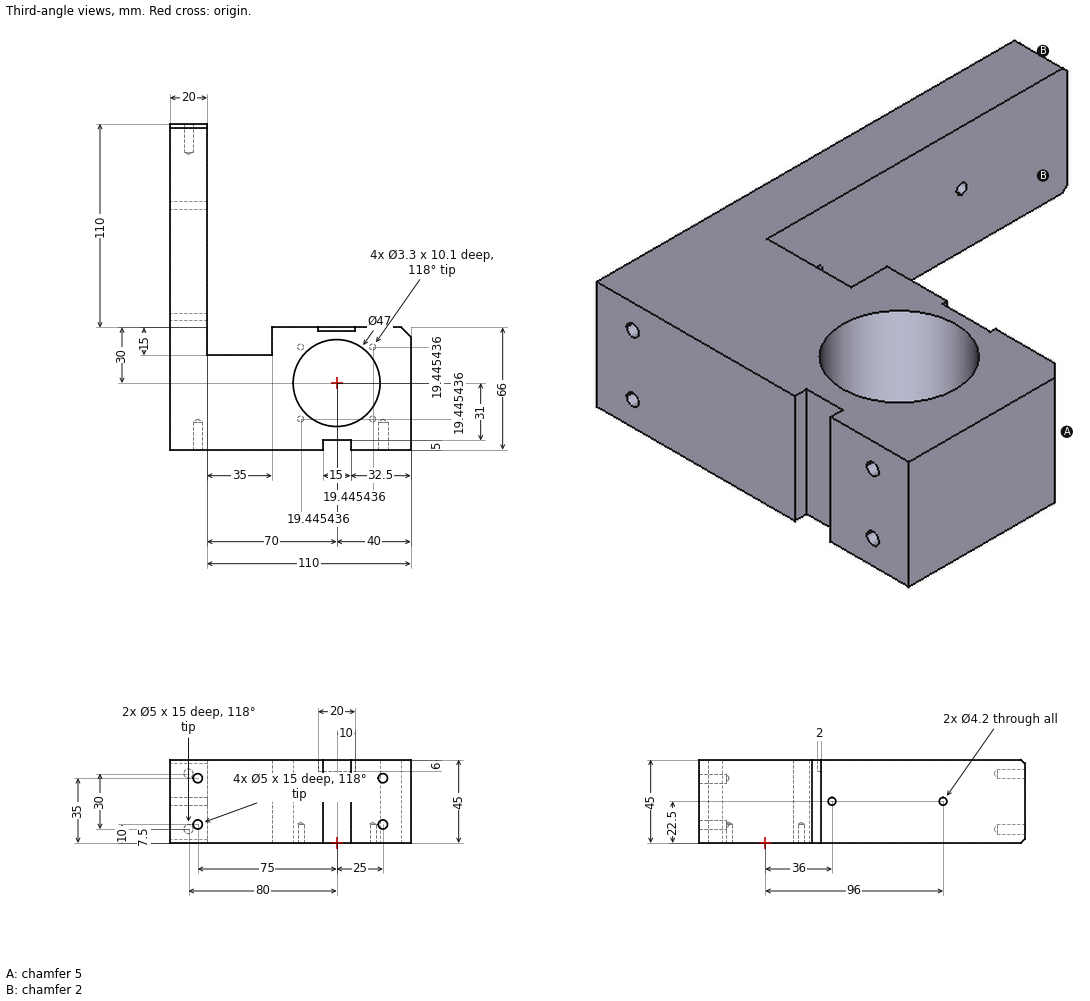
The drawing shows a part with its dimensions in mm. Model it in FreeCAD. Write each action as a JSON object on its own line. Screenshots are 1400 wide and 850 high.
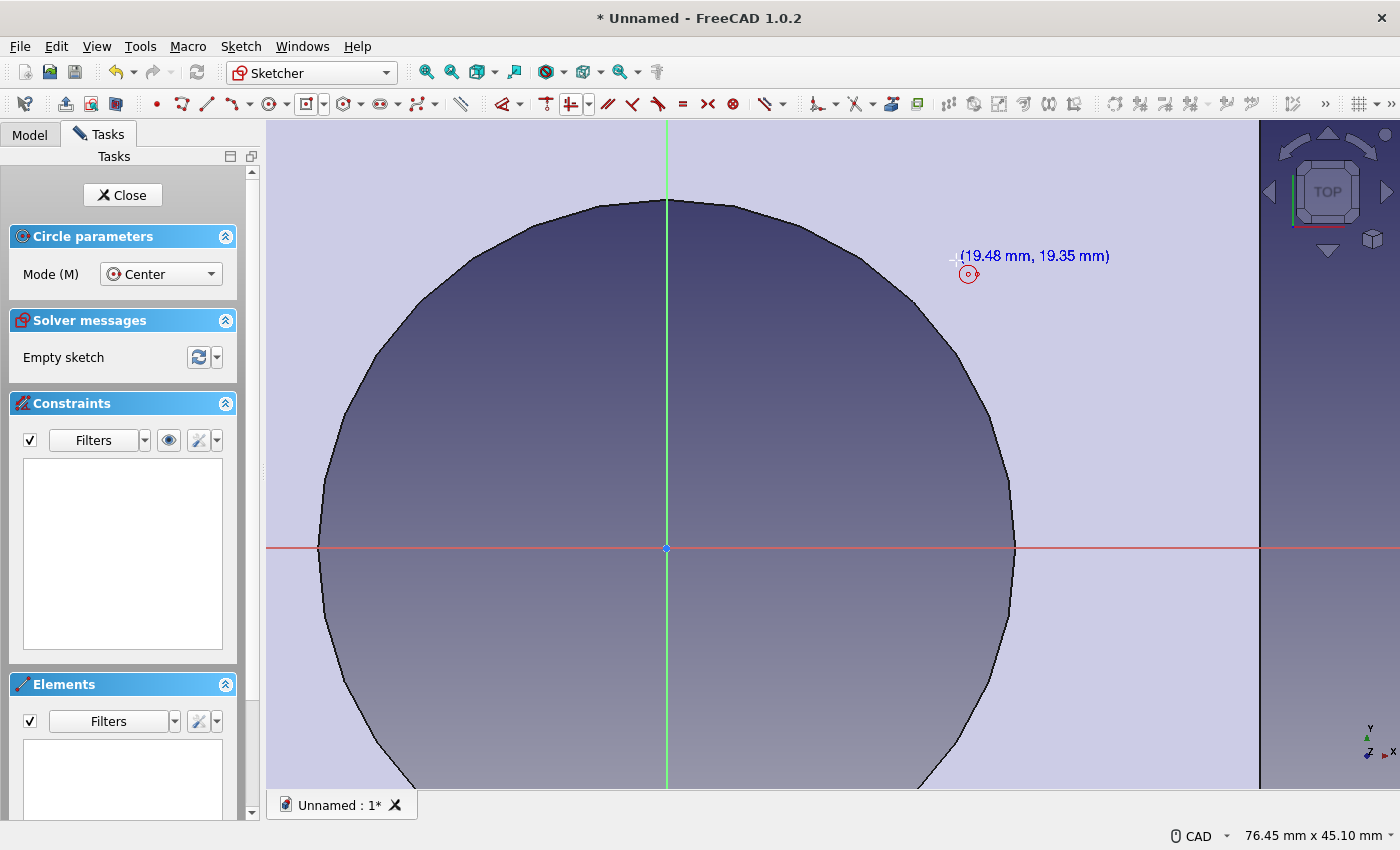
{"action": "left_click", "coordinate": [955, 260]}
{"action": "left_click", "coordinate": [972, 243]}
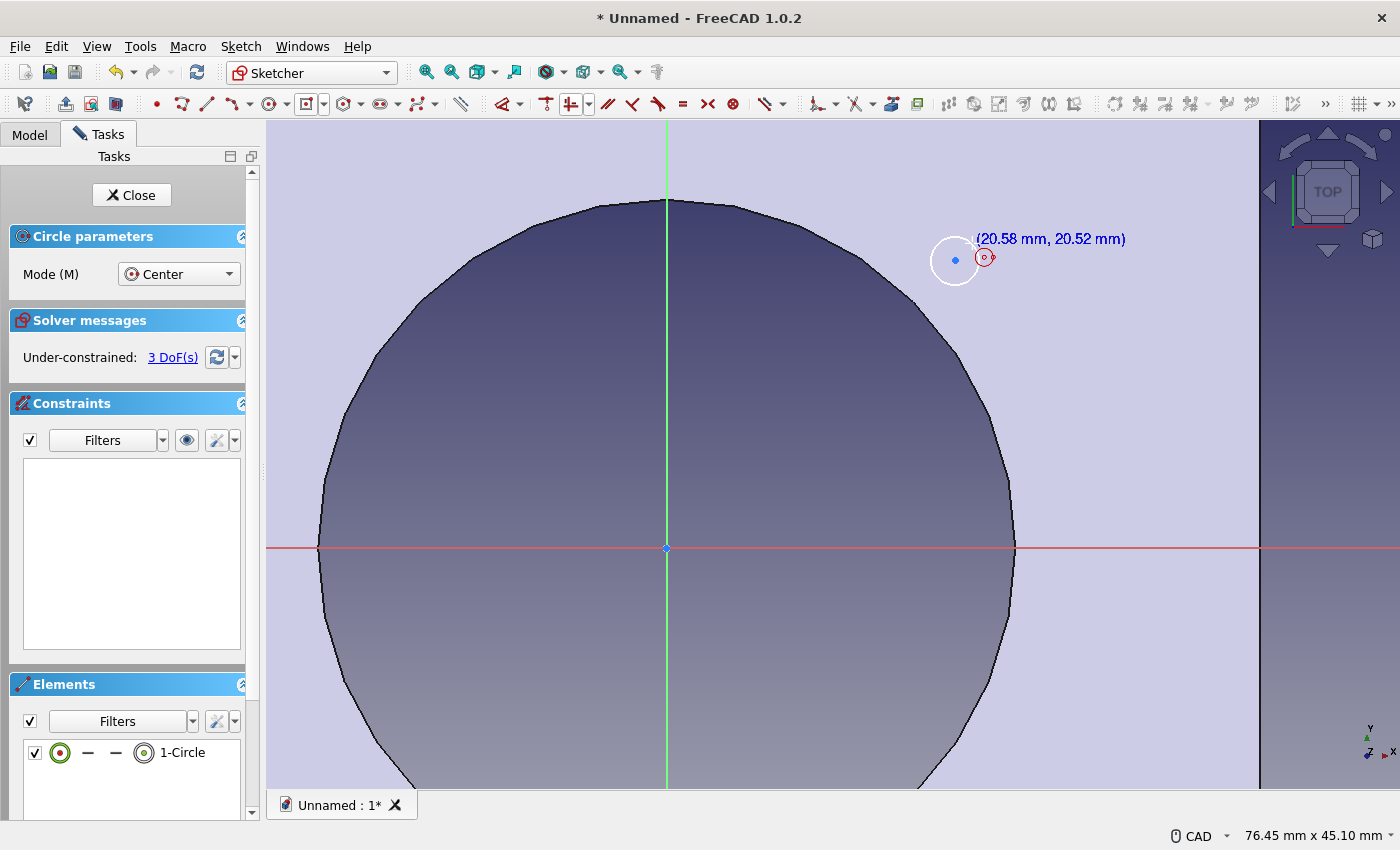
{"action": "scroll", "coordinate": [963, 264], "scroll_direction": "down", "scroll_amount": 2}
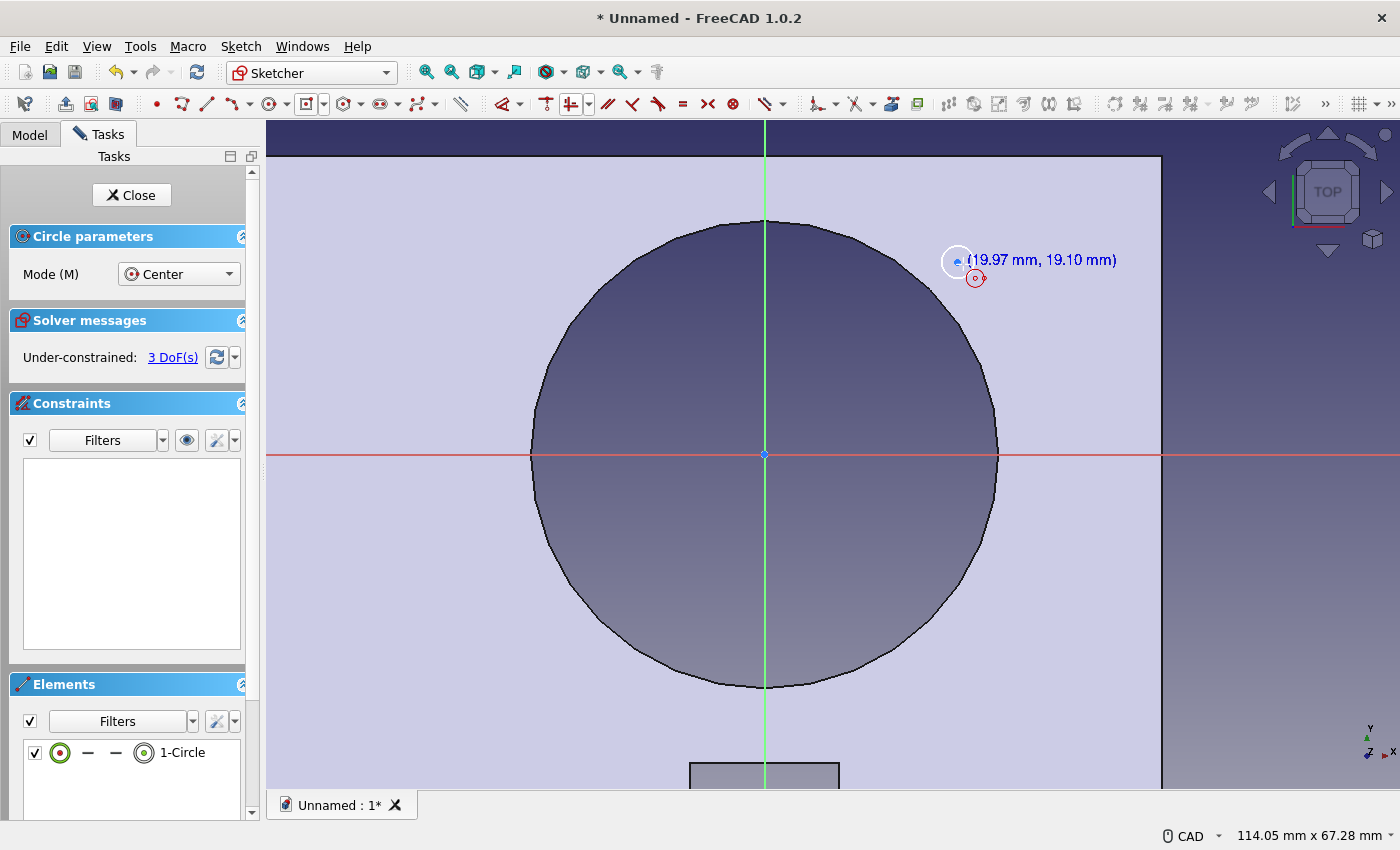
{"action": "scroll", "coordinate": [571, 648], "scroll_direction": "up", "scroll_amount": 2}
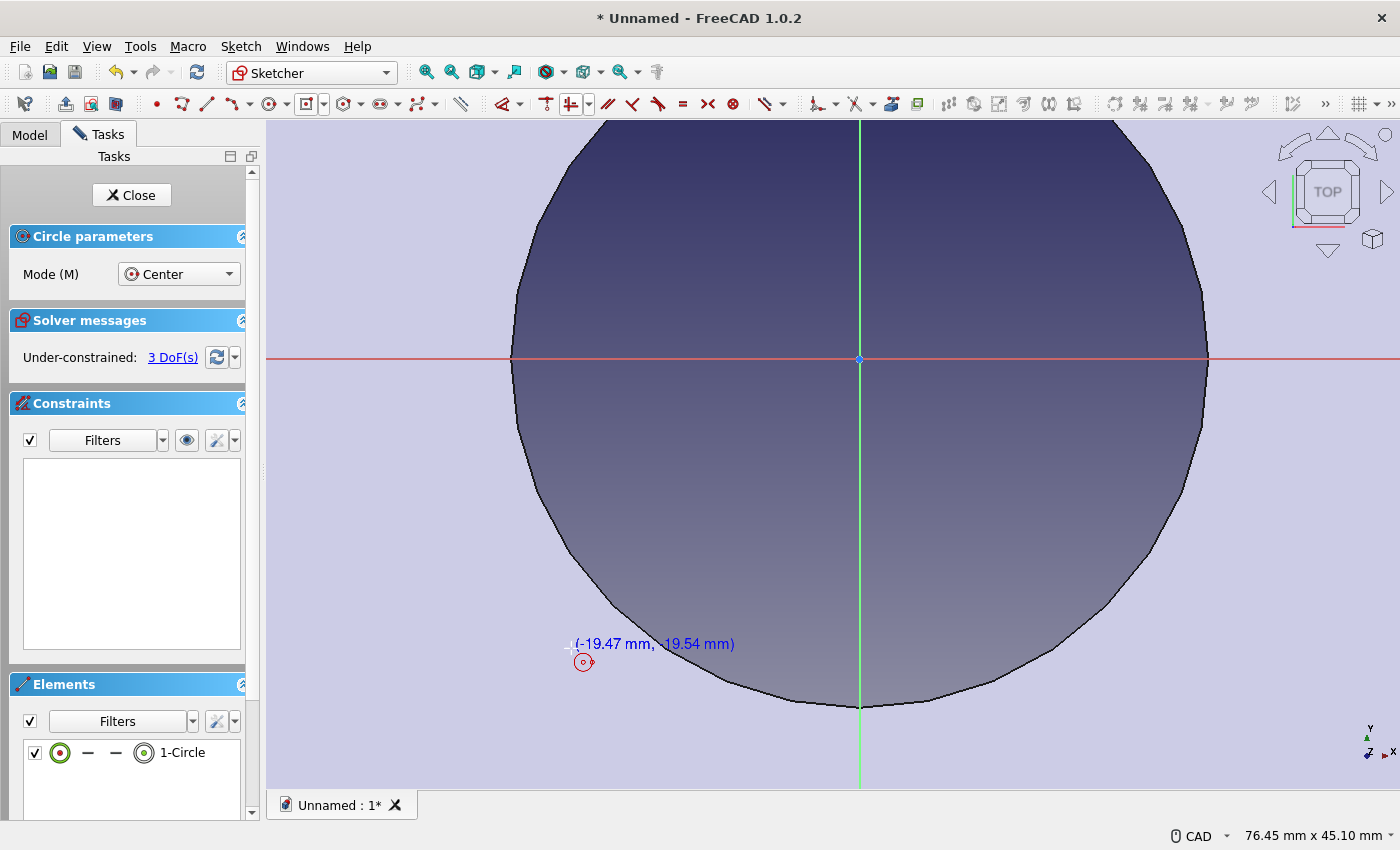
{"action": "left_click", "coordinate": [571, 648]}
{"action": "left_click", "coordinate": [589, 630]}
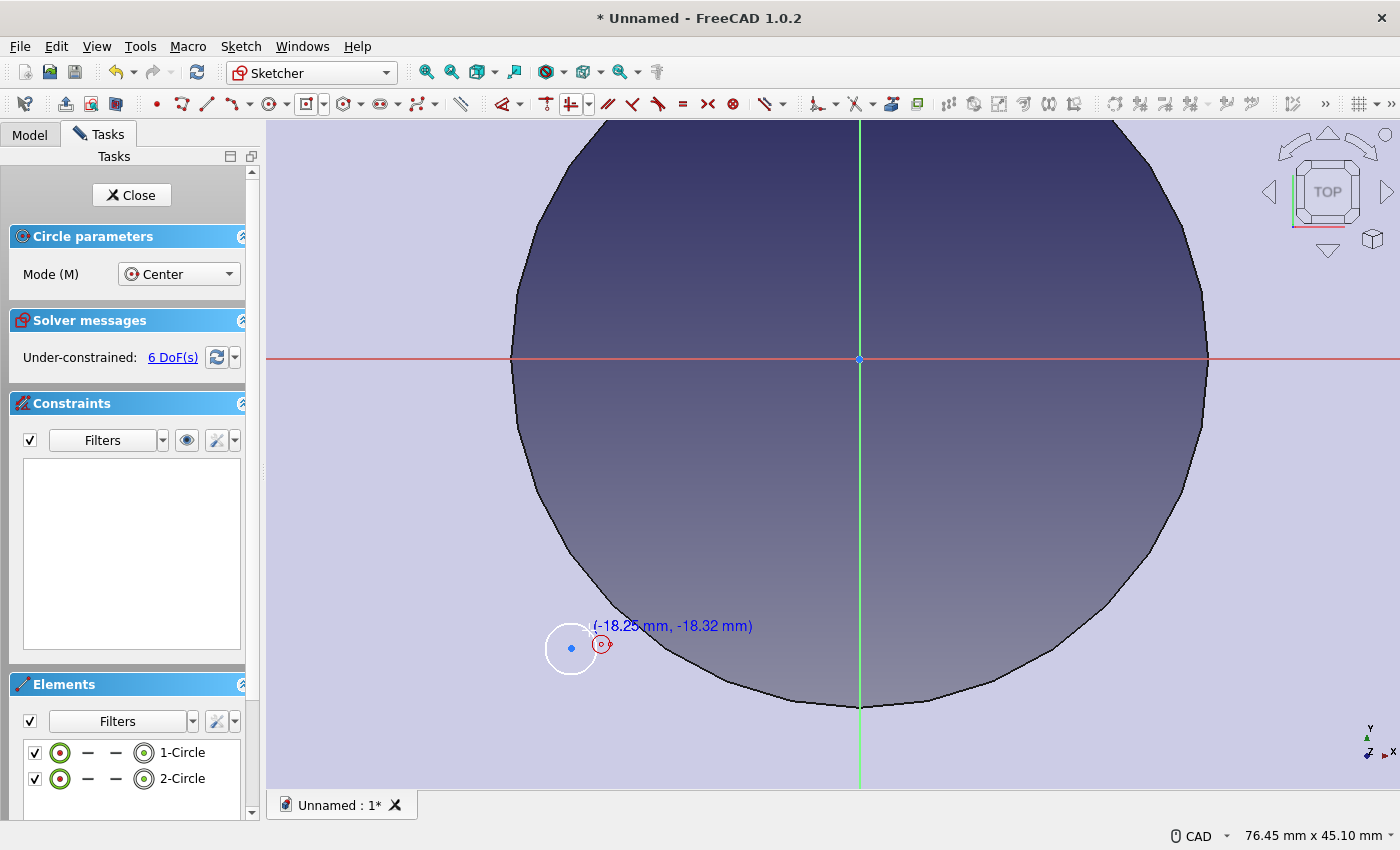
{"action": "left_click", "coordinate": [1148, 648]}
{"action": "left_click", "coordinate": [1165, 630]}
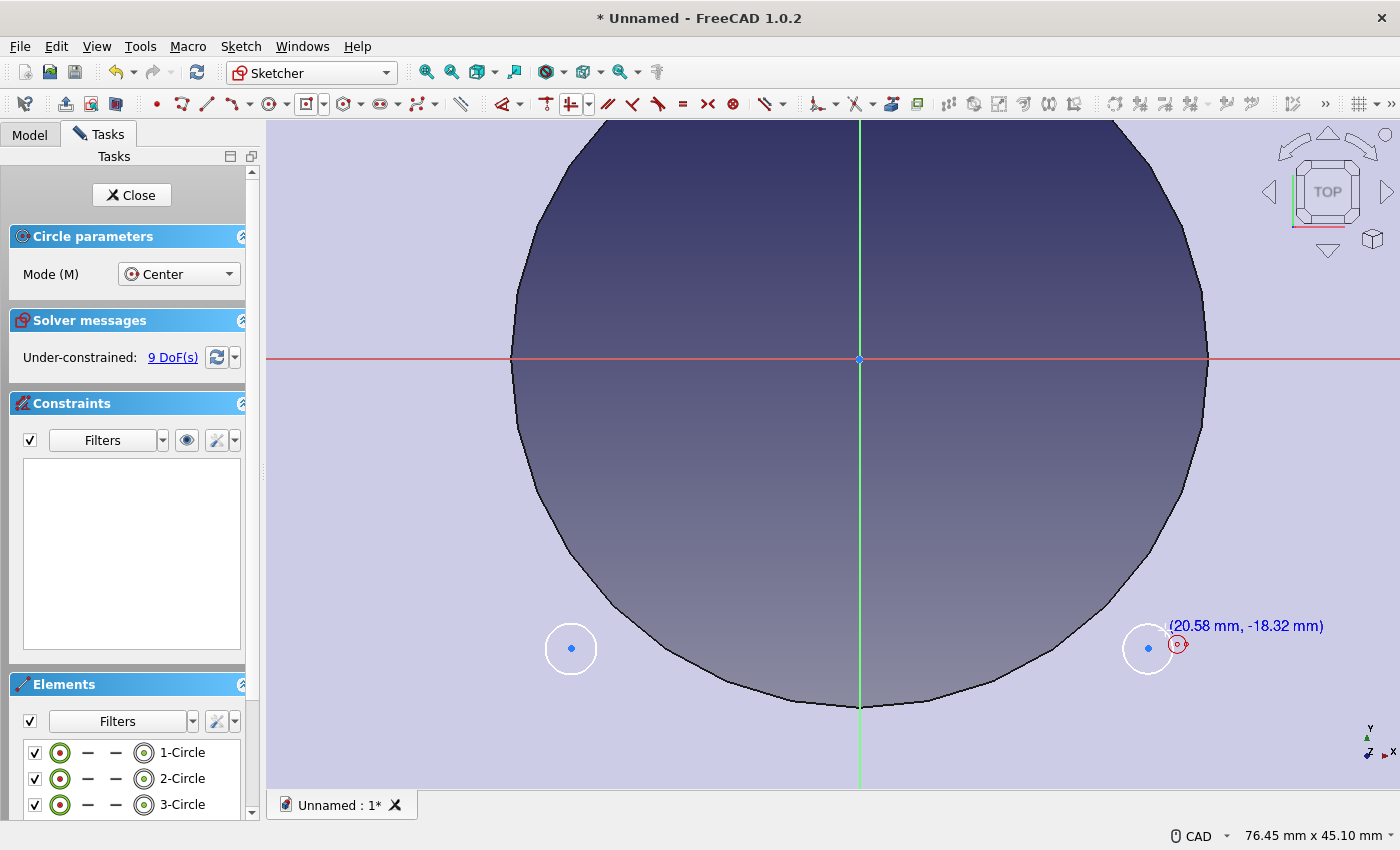
{"action": "scroll", "coordinate": [571, 648], "scroll_direction": "down", "scroll_amount": 2}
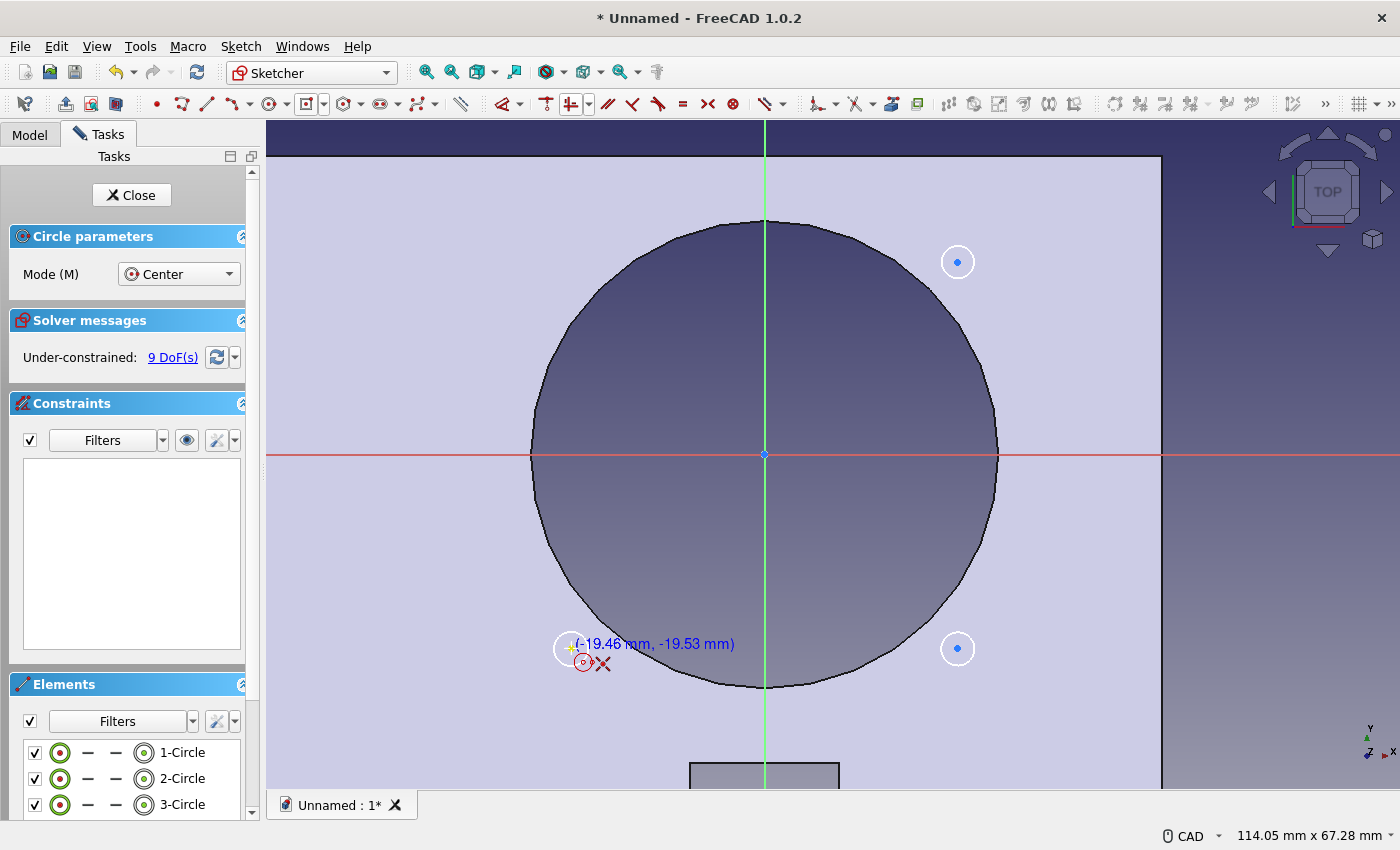
{"action": "scroll", "coordinate": [571, 261], "scroll_direction": "up", "scroll_amount": 2}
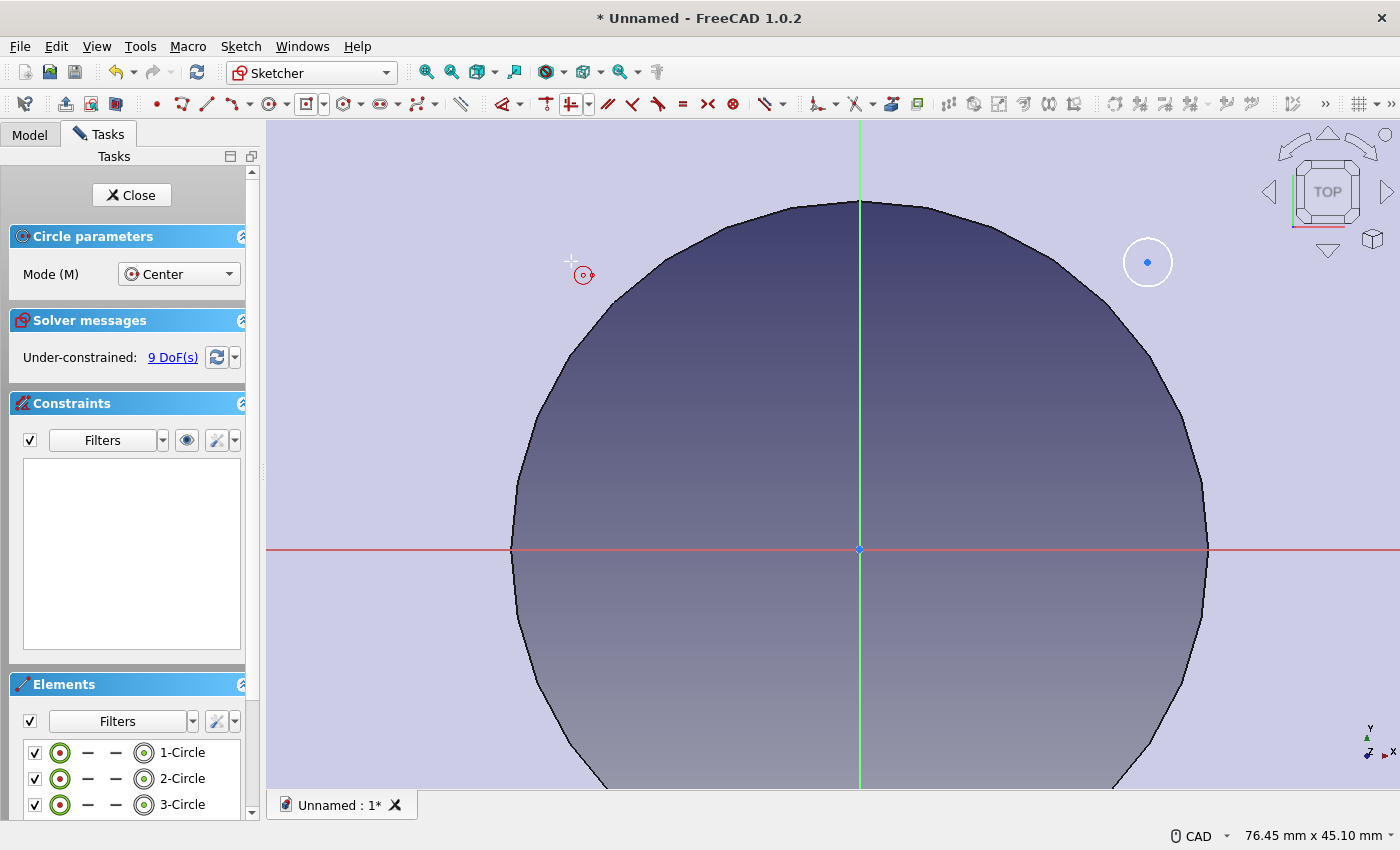
{"action": "left_click", "coordinate": [571, 261]}
{"action": "left_click", "coordinate": [589, 244]}
{"action": "key", "text": "Escape"}